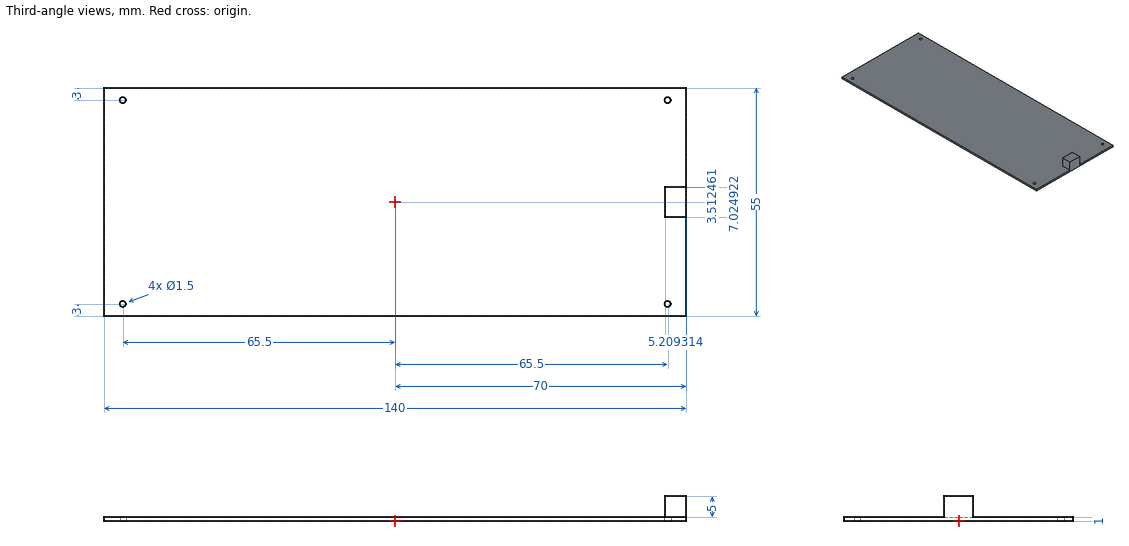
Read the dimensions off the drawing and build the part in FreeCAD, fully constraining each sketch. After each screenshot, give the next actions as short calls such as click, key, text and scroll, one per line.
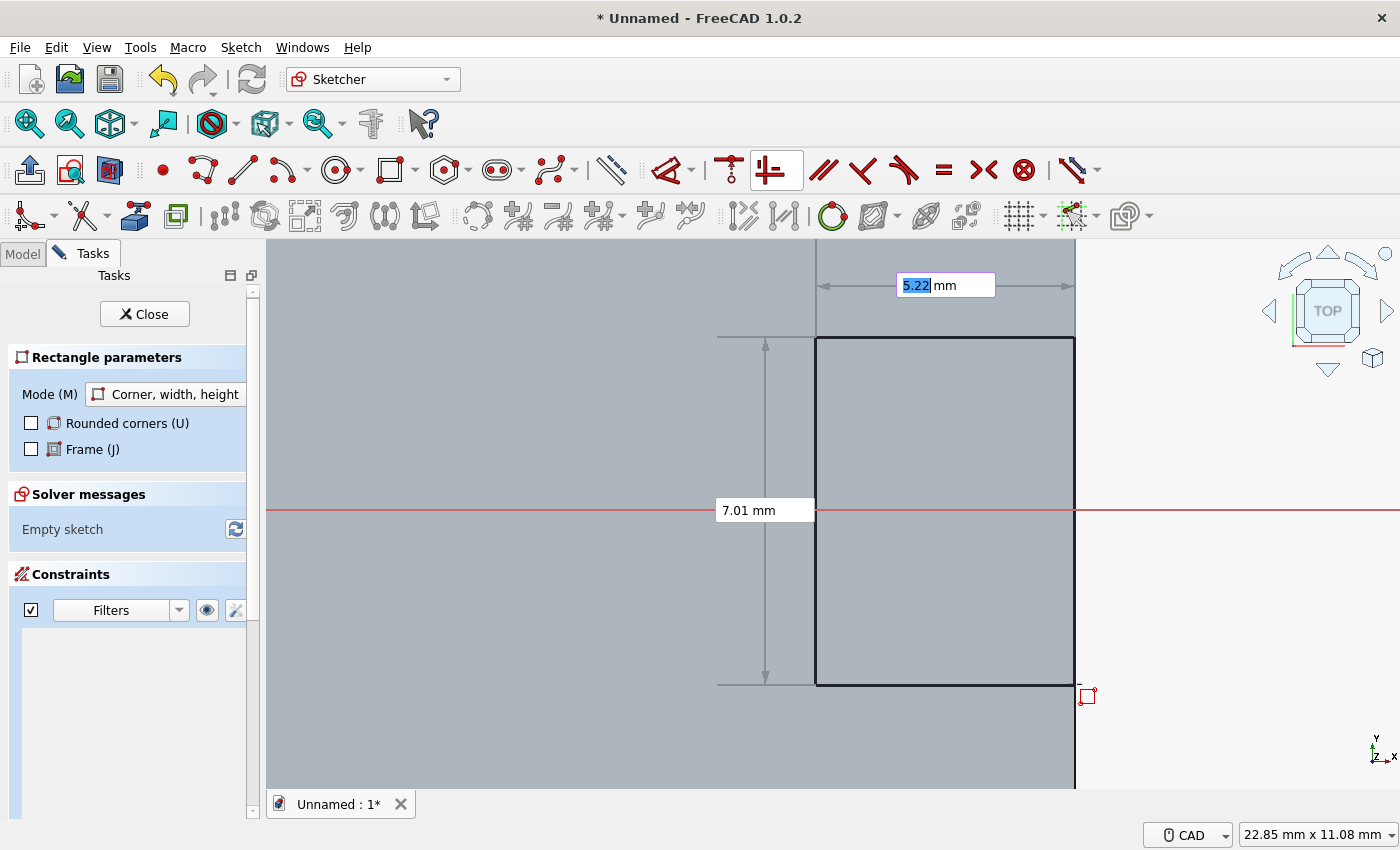
text(5.209314)
key(Tab)
text(7.024922)
key(Return)
key(Escape)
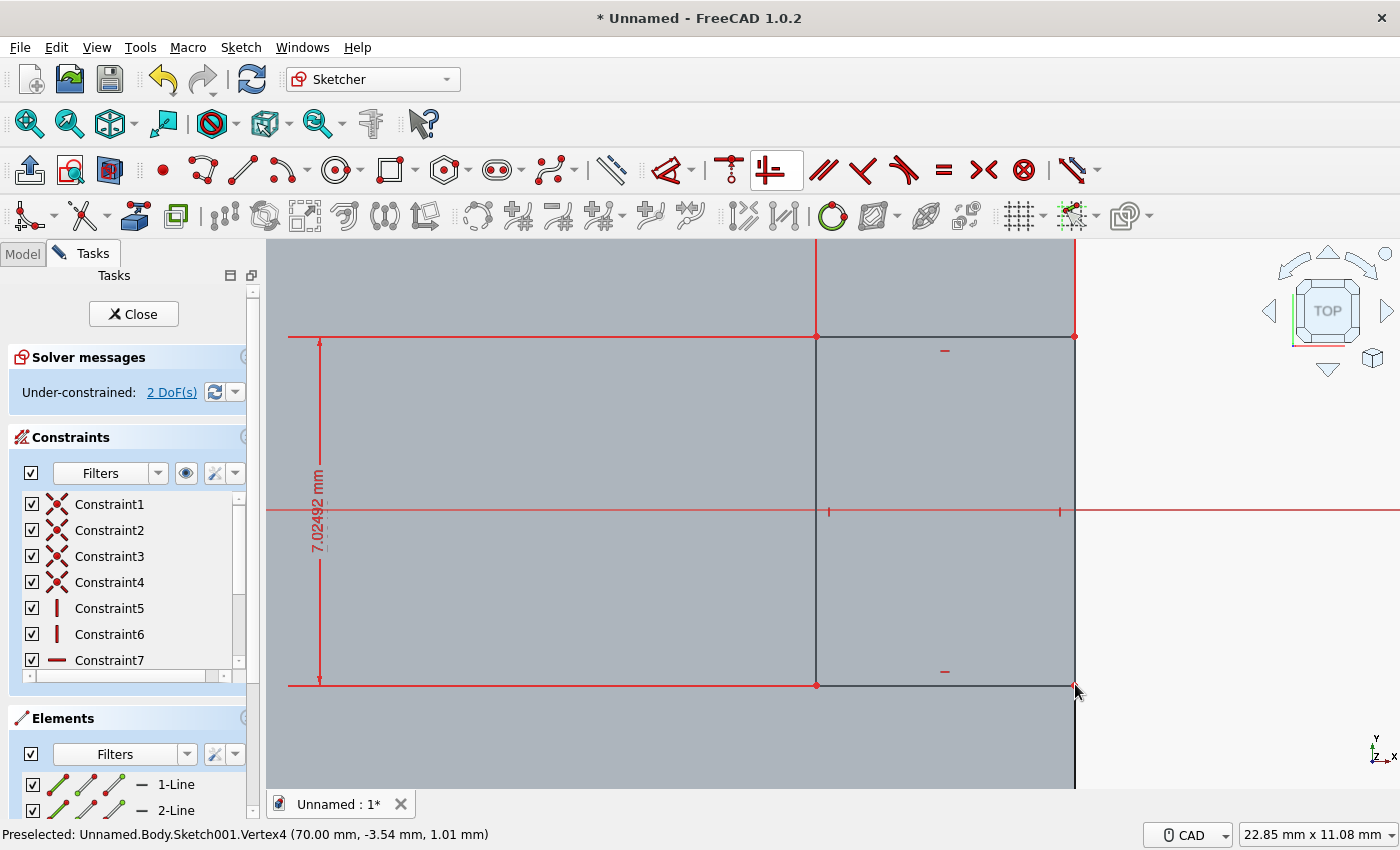
click(666, 170)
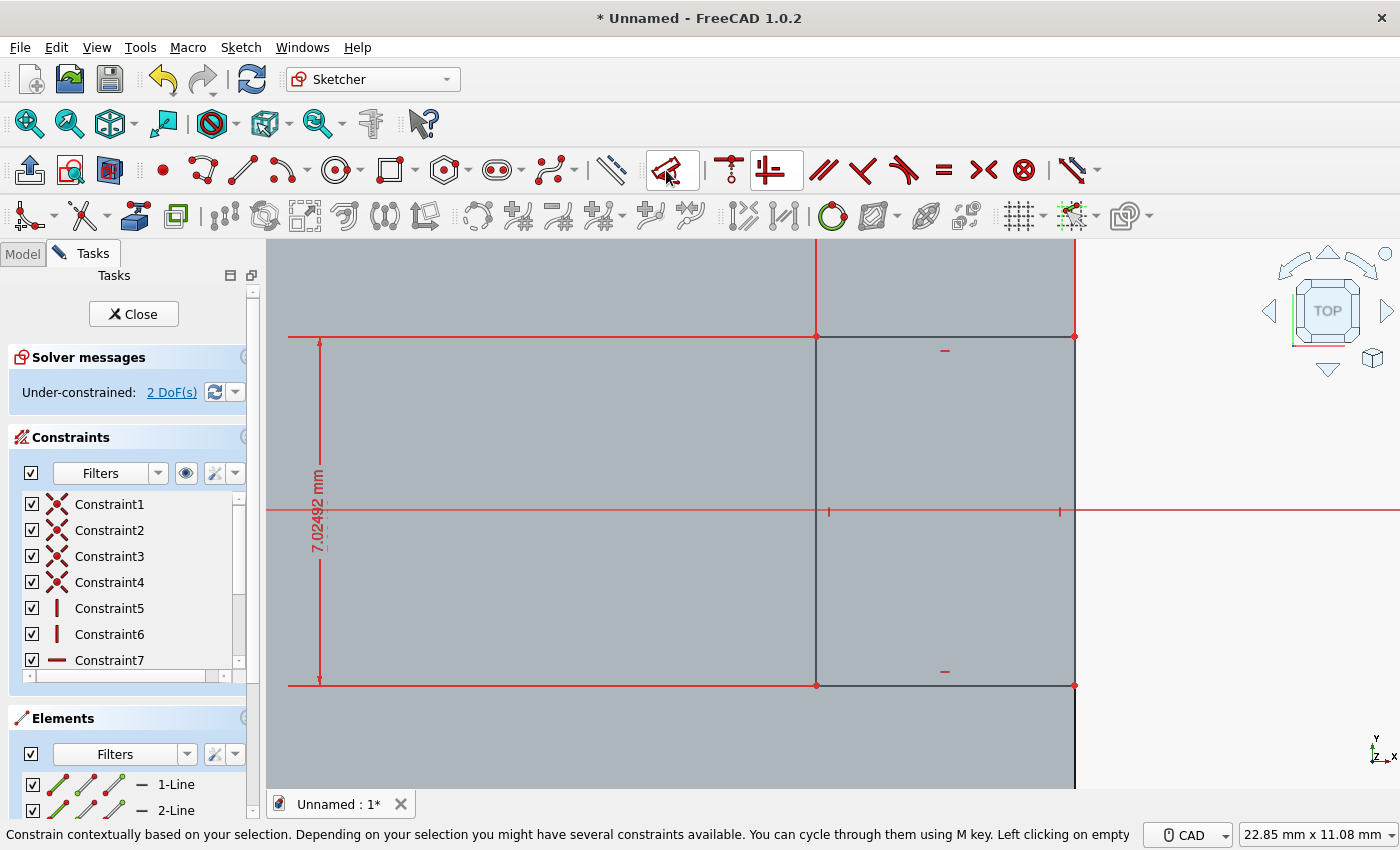
click(1075, 686)
click(684, 720)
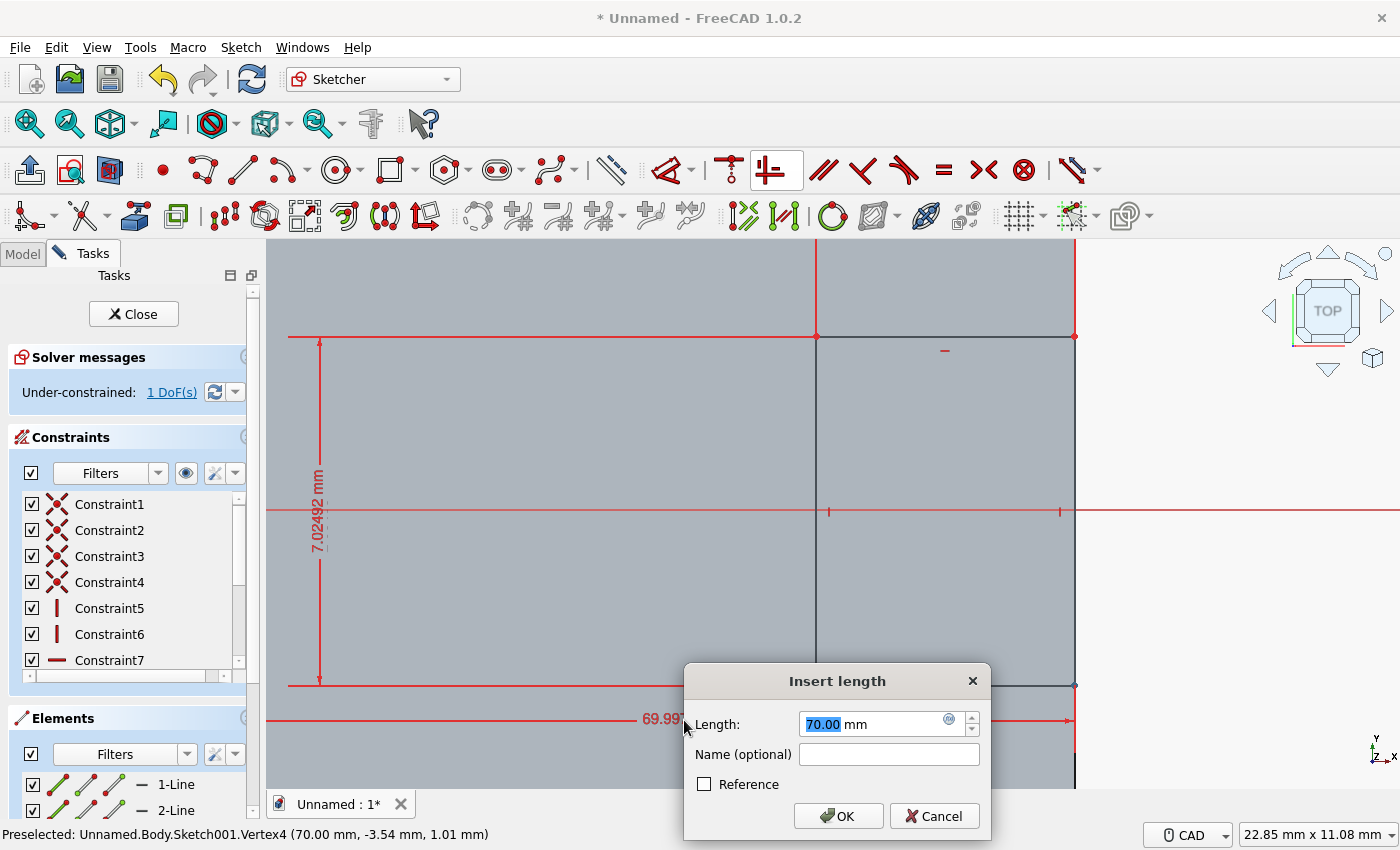
text(70)
key(Return)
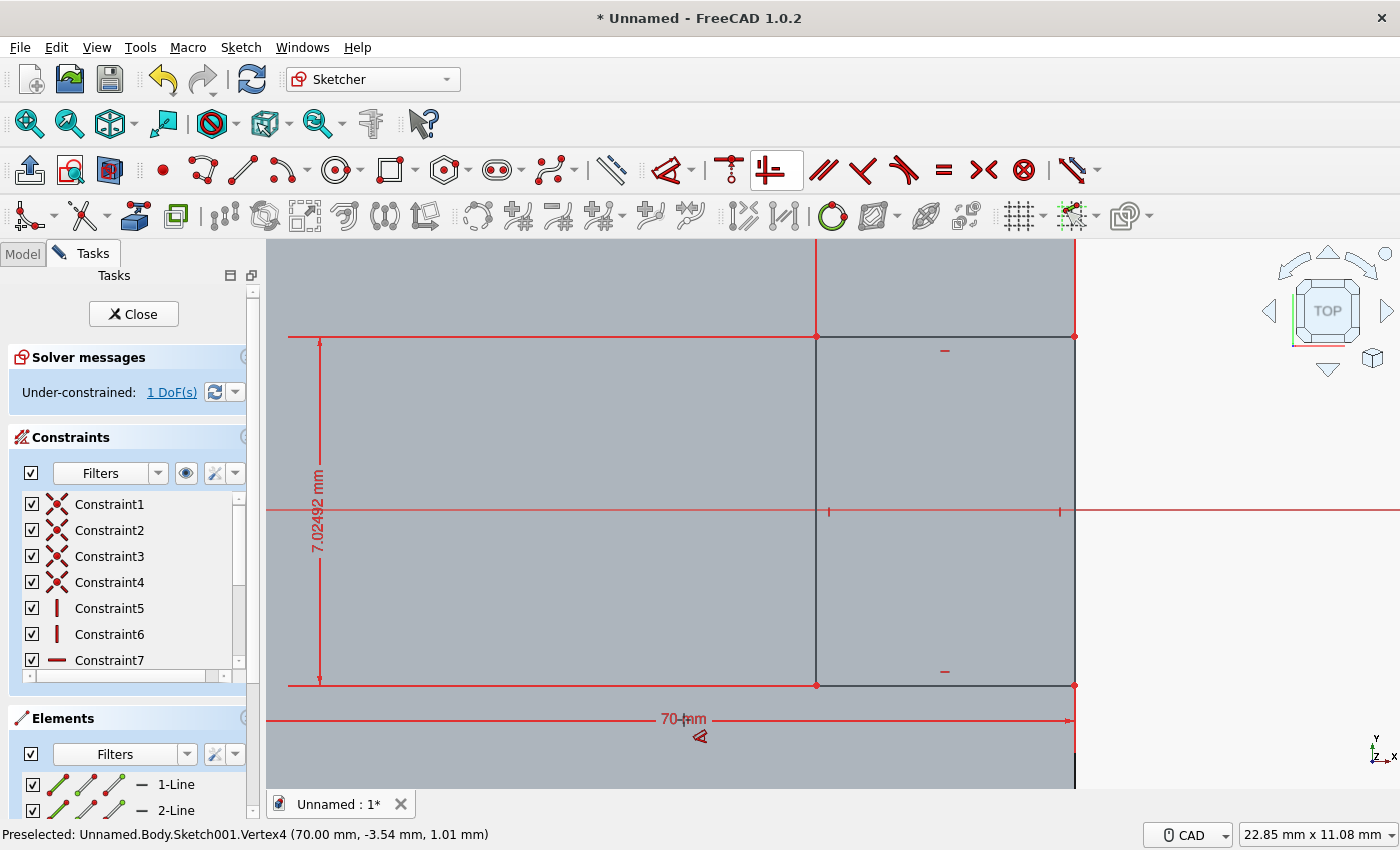
click(816, 337)
click(850, 423)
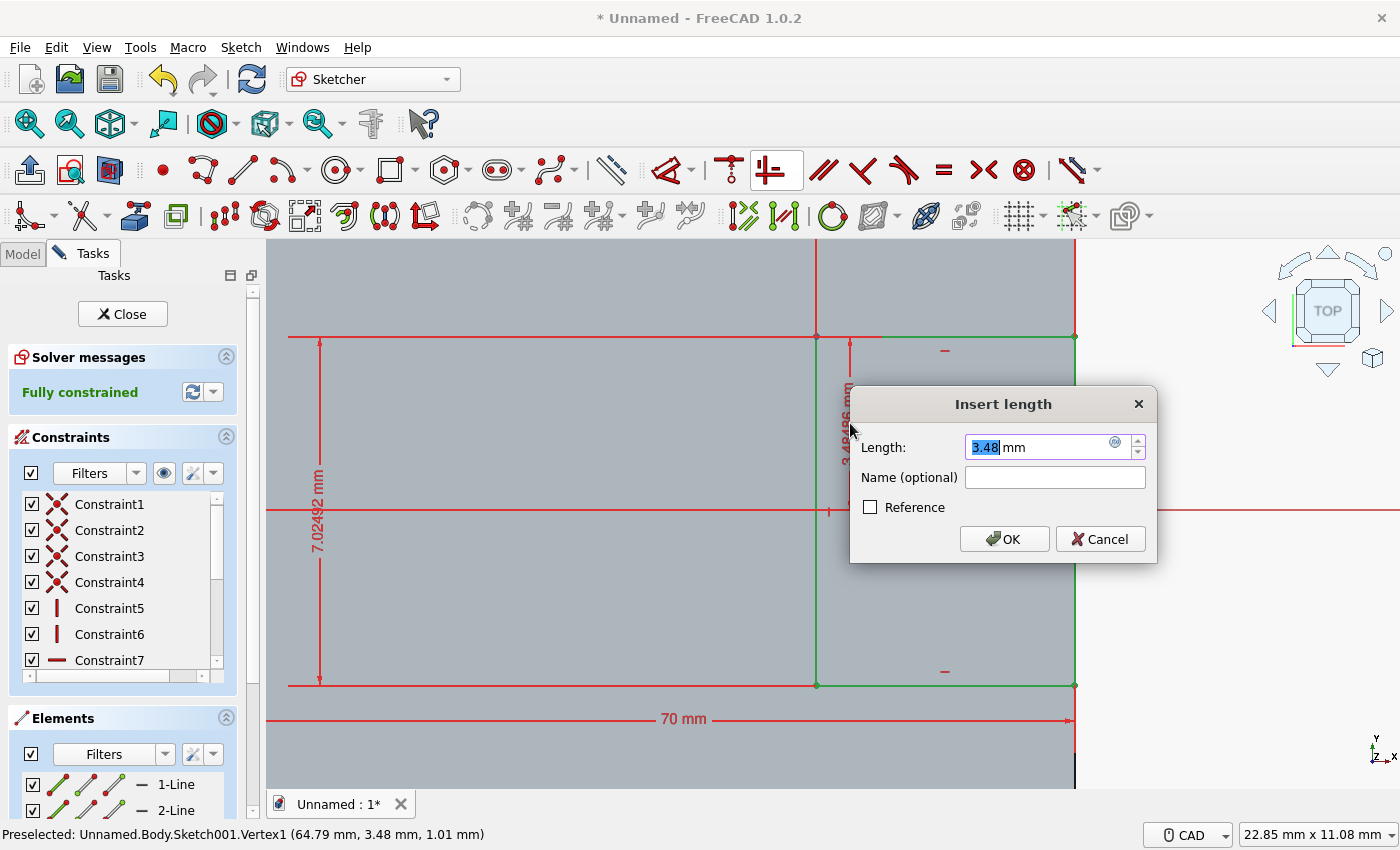
text(3.512461)
key(Return)
key(Escape)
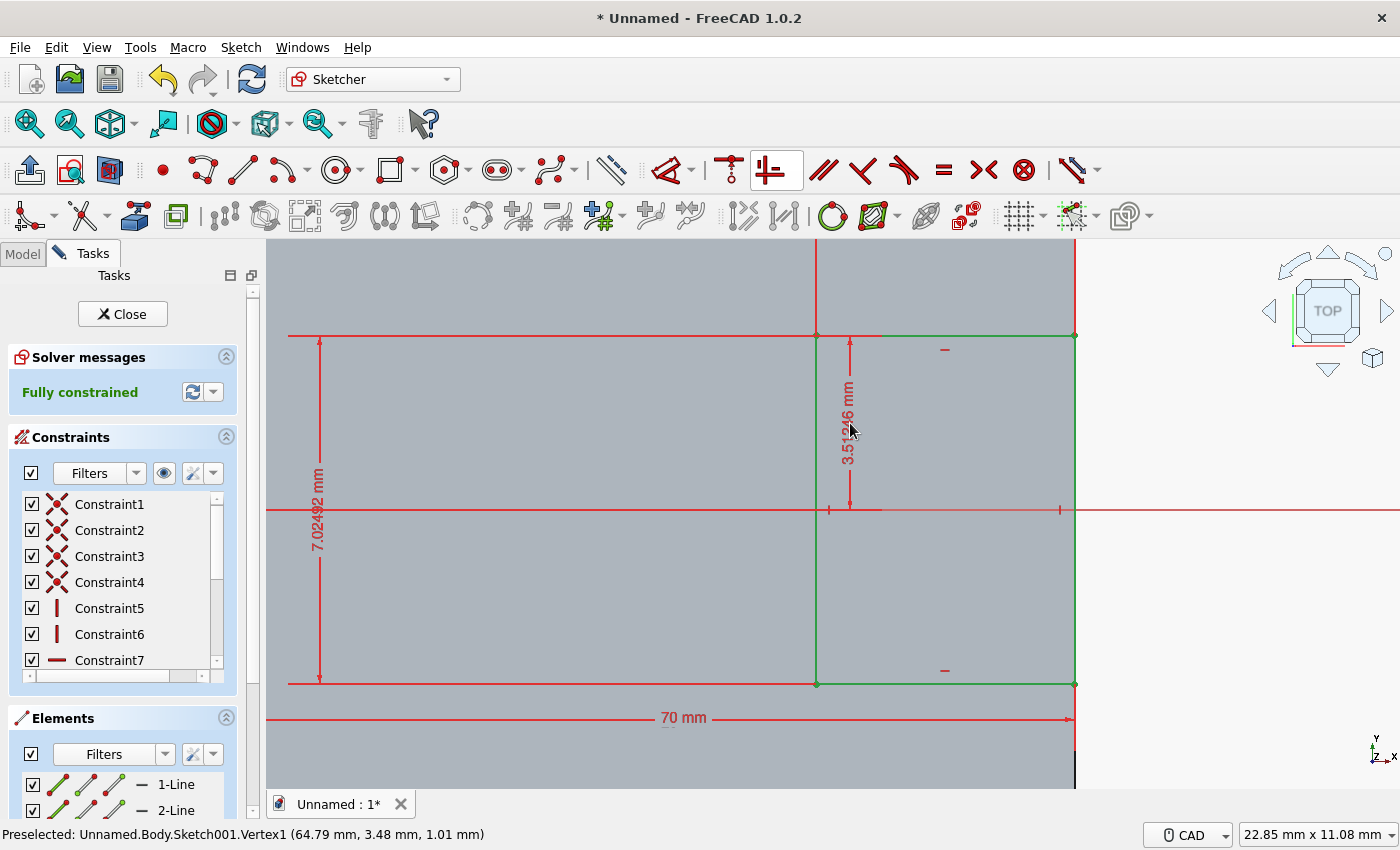
click(123, 314)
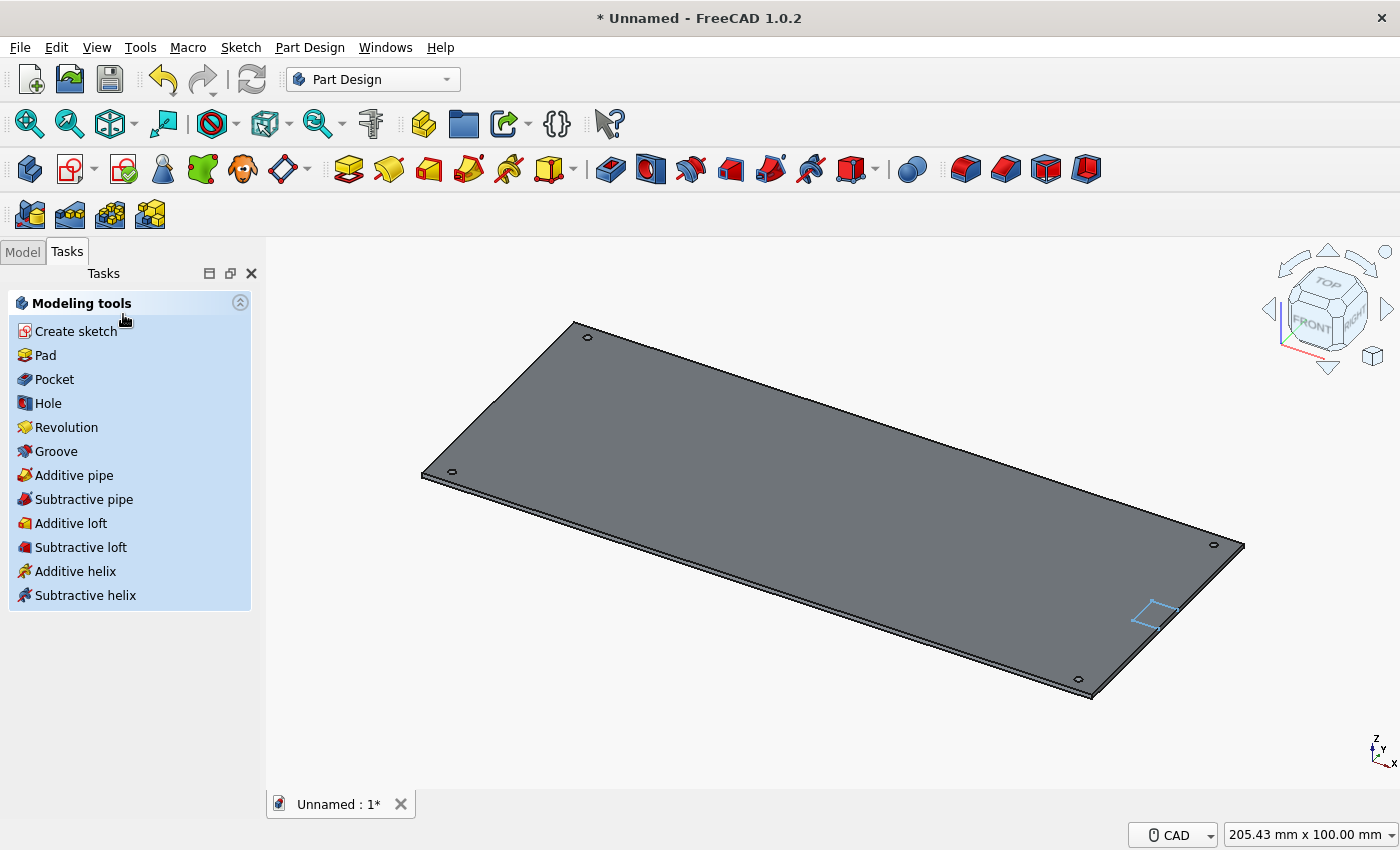
click(350, 170)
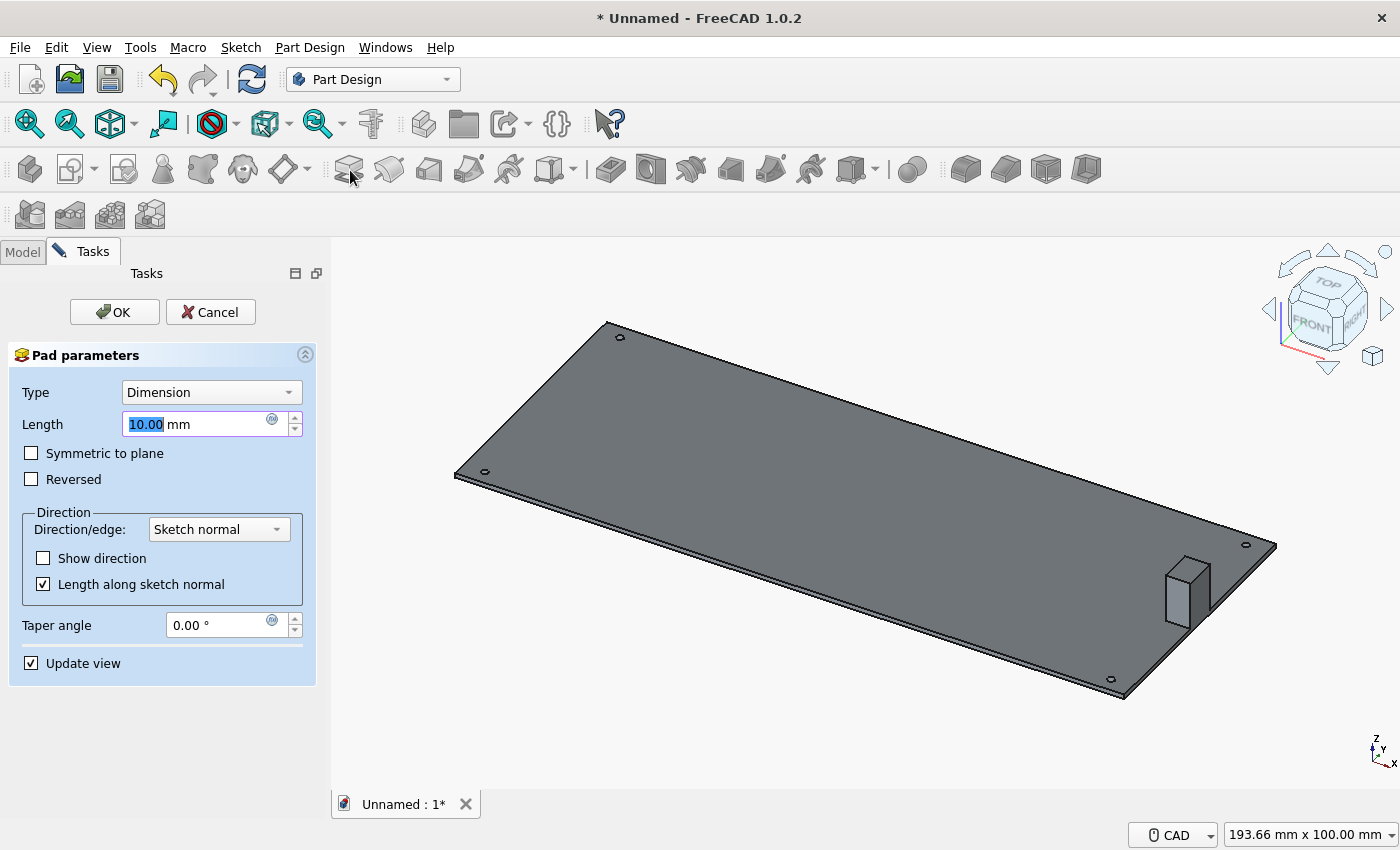
text(5)
key(Tab)